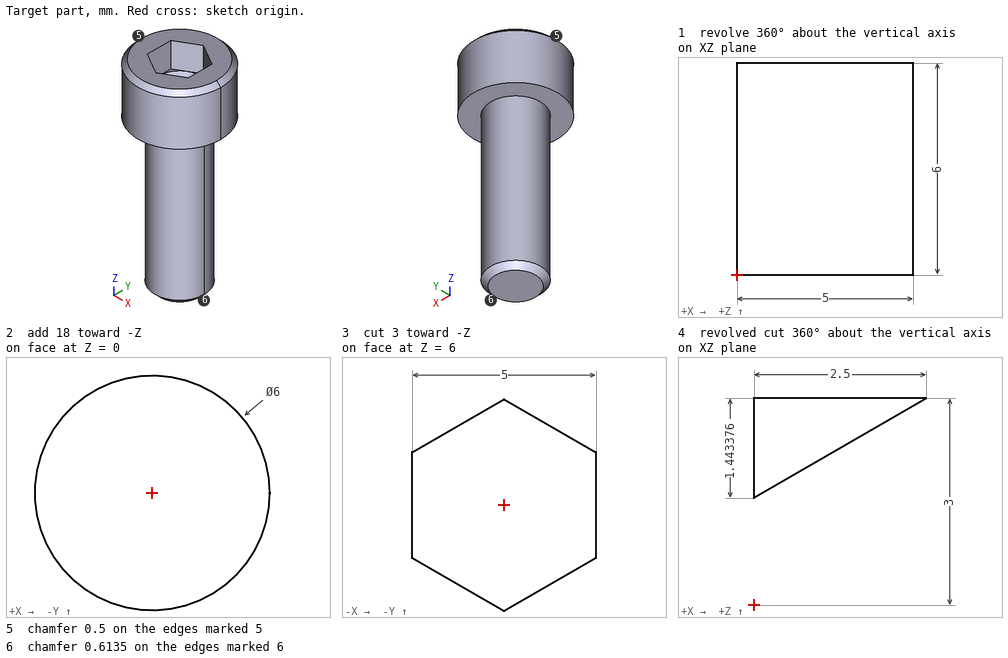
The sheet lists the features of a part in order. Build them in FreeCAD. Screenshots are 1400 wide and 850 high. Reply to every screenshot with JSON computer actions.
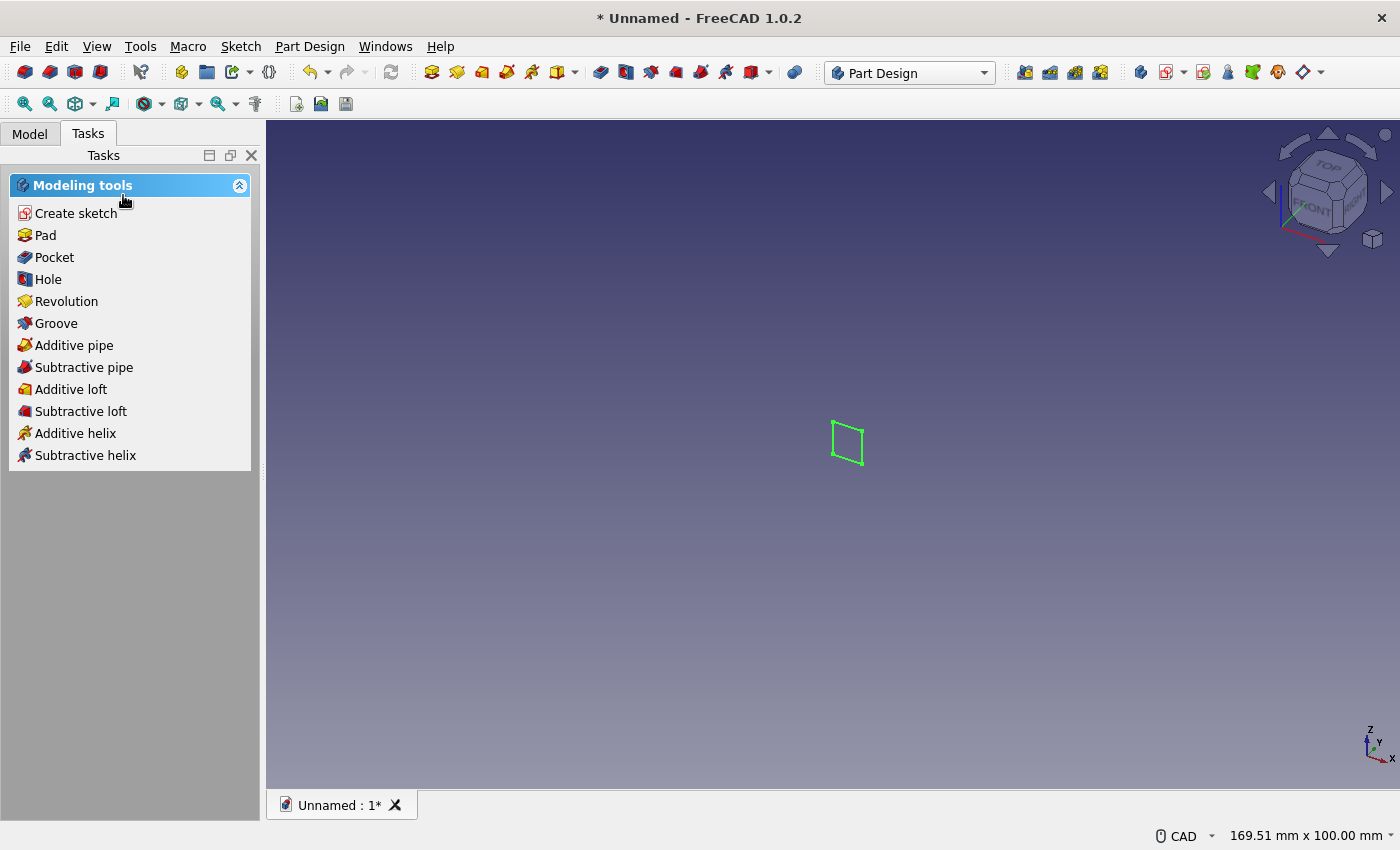
{"action": "left_click", "coordinate": [457, 72]}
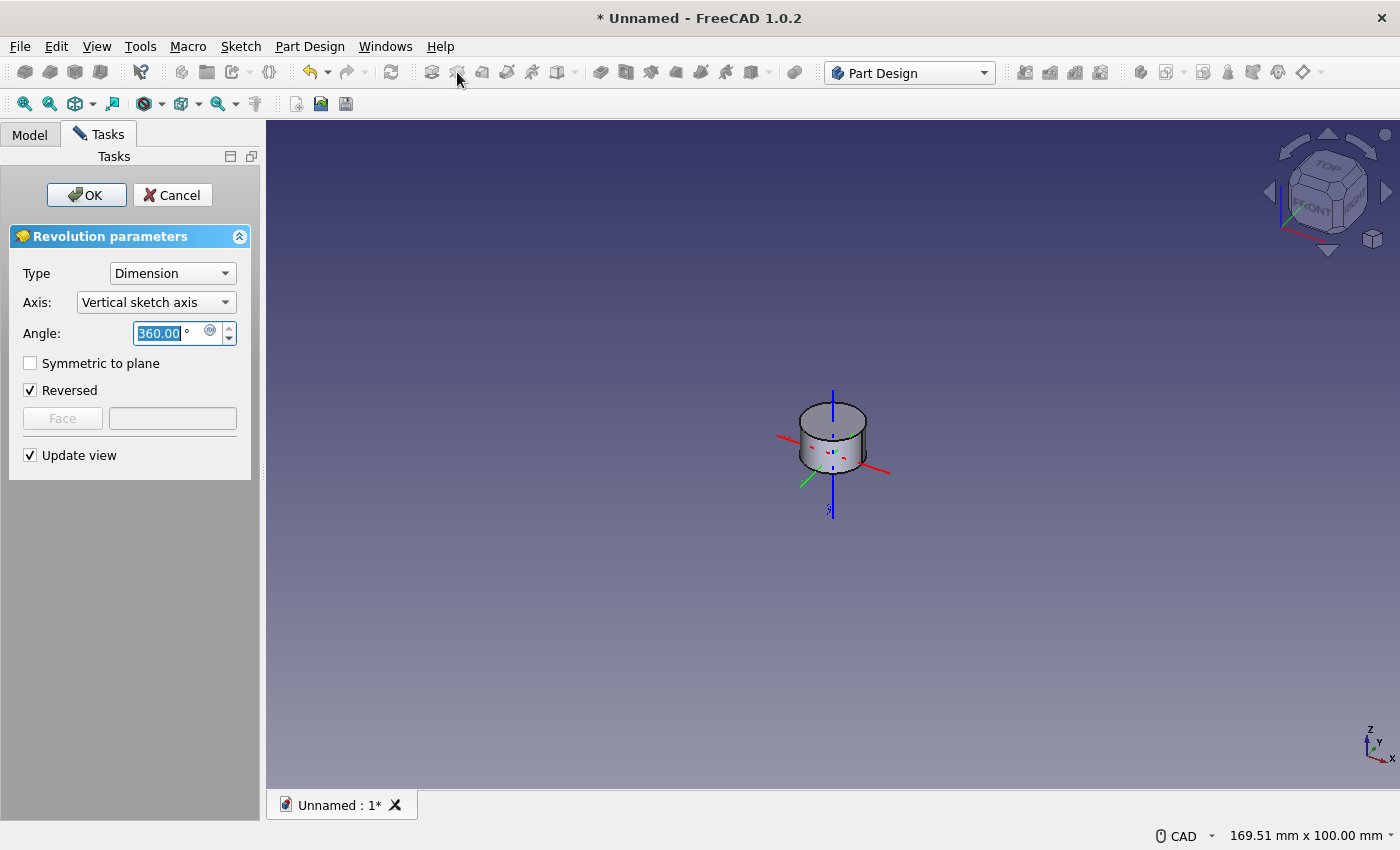
{"action": "left_click", "coordinate": [87, 195]}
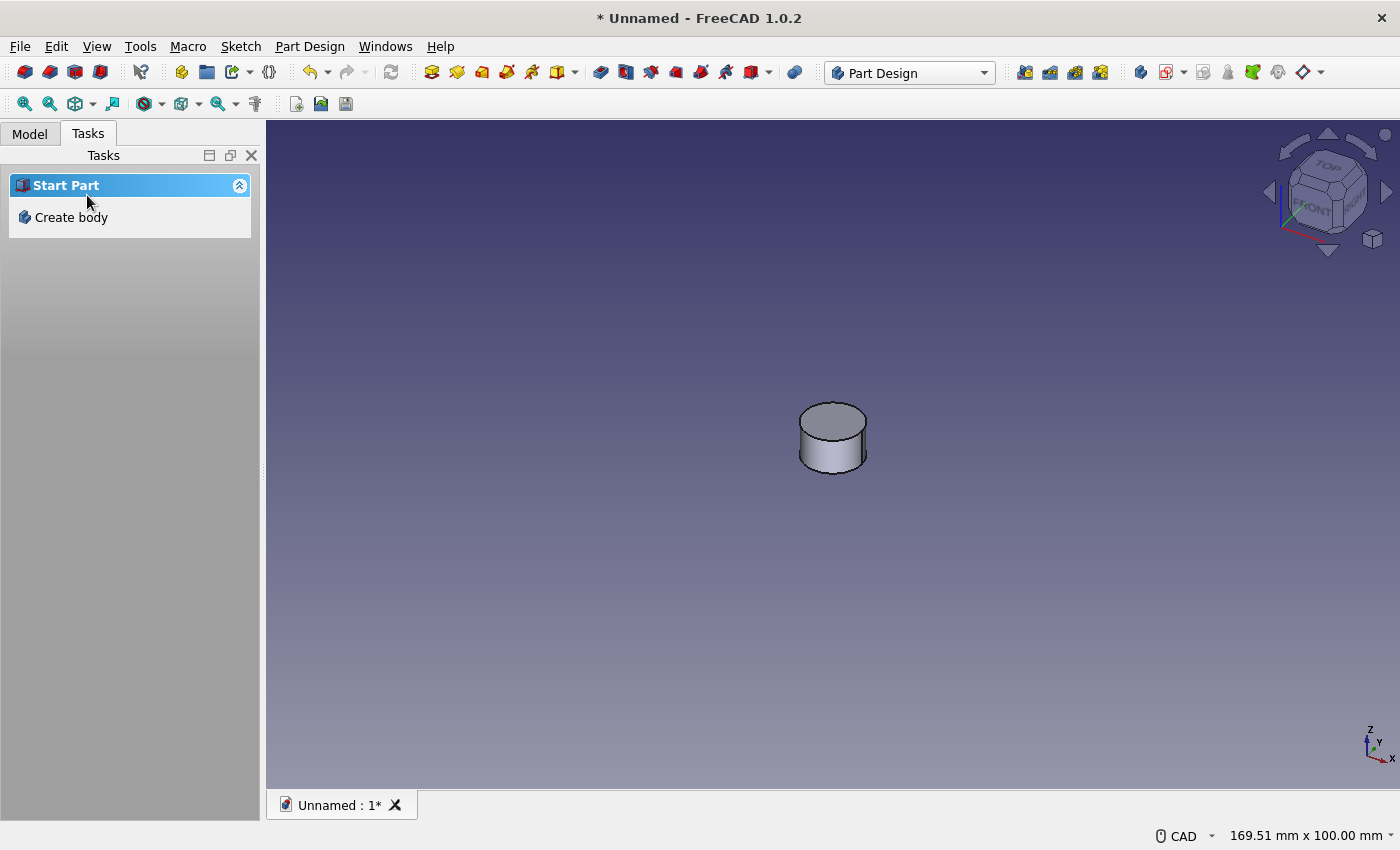
{"action": "left_click", "coordinate": [25, 104]}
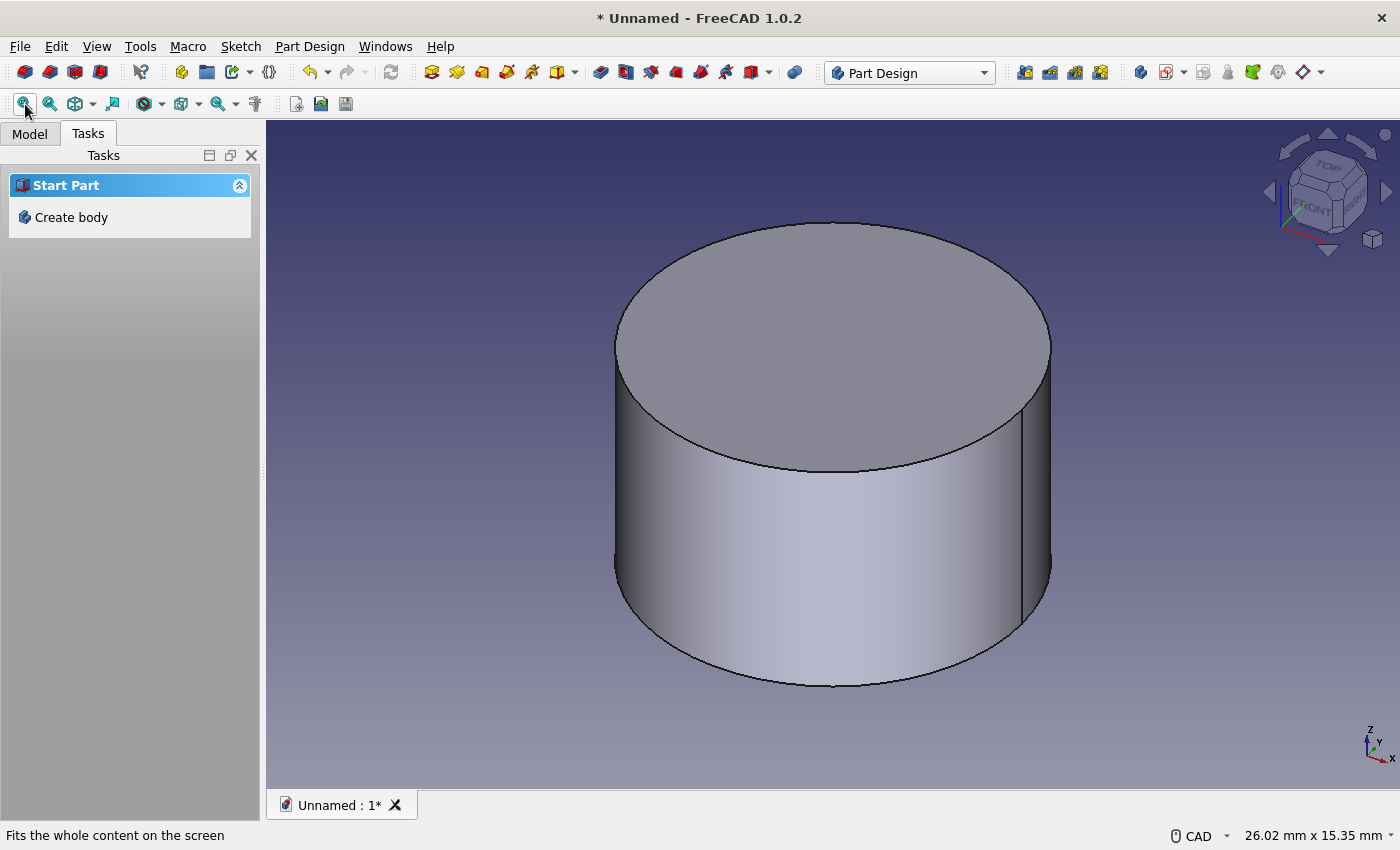
{"action": "key", "text": "5"}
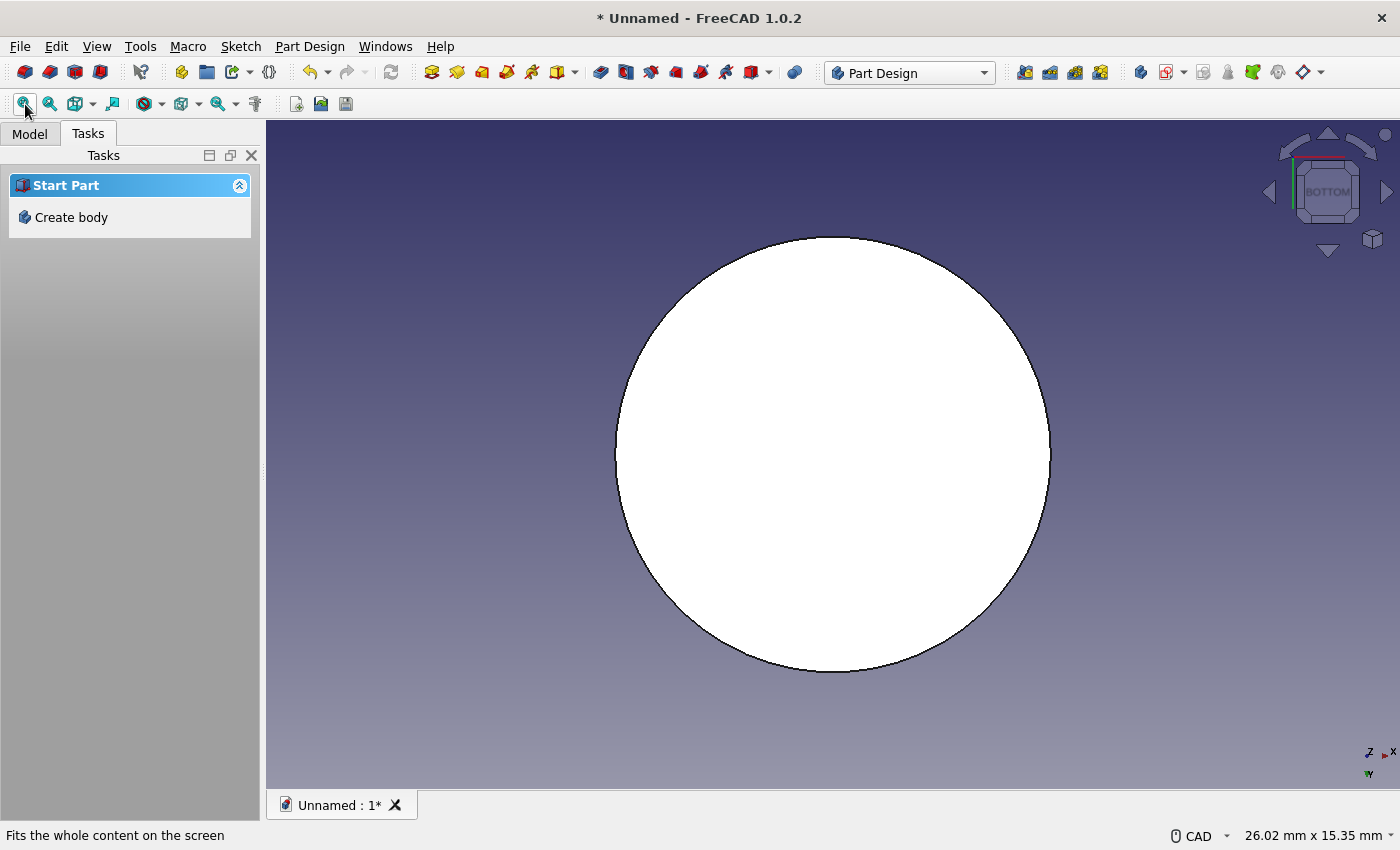
{"action": "left_click", "coordinate": [833, 454]}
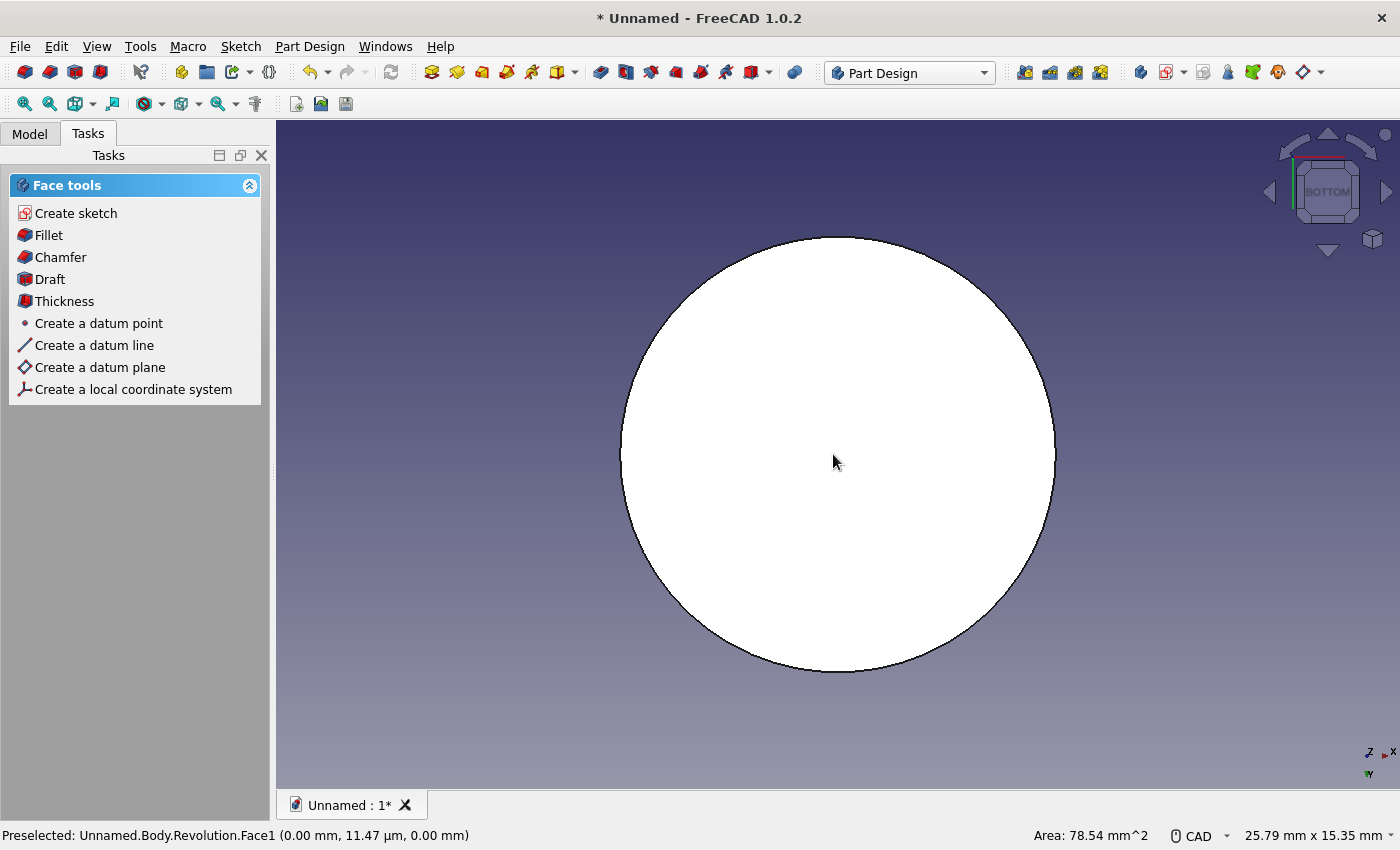
{"action": "left_click", "coordinate": [1166, 72]}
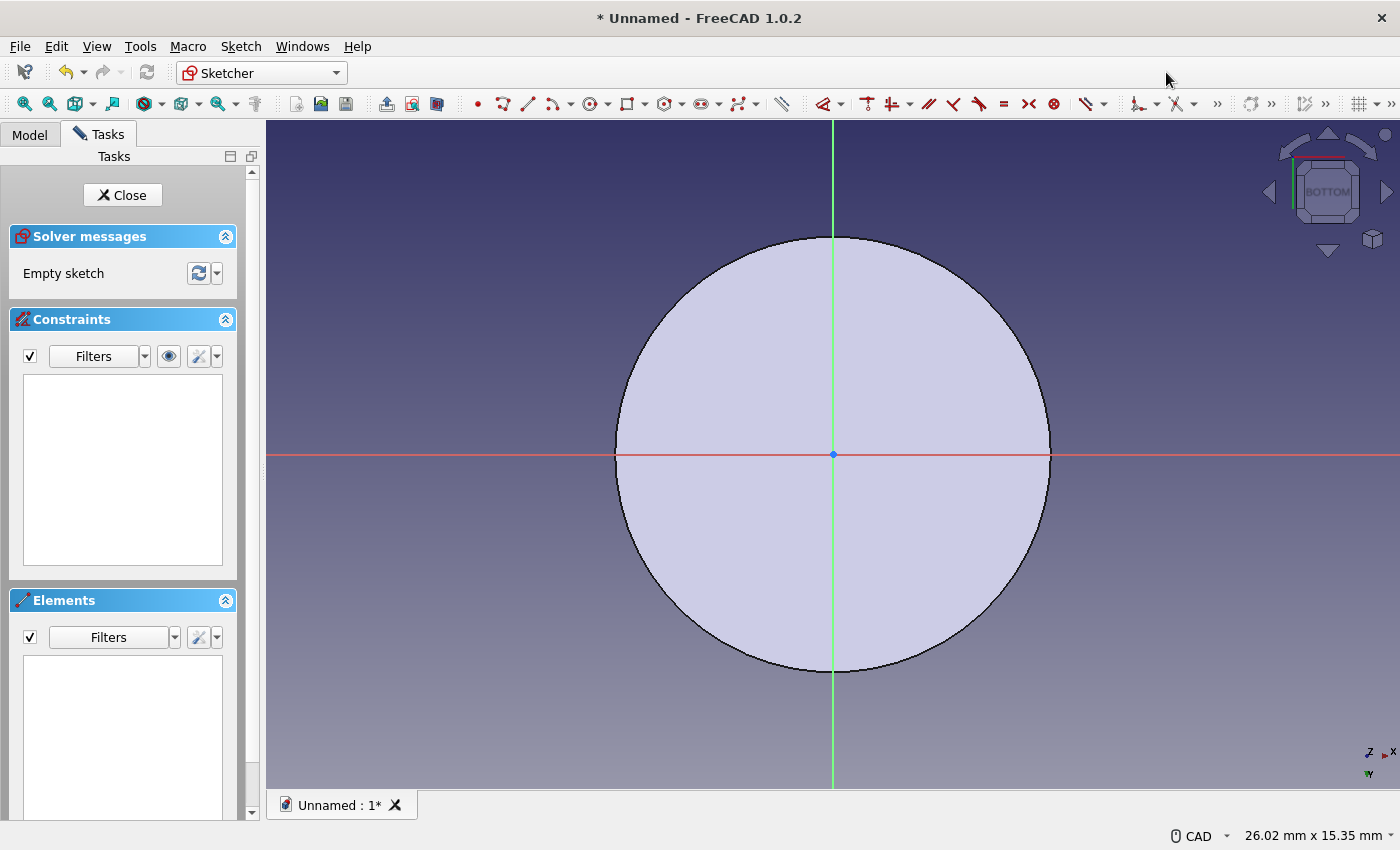
{"action": "scroll", "coordinate": [916, 455], "scroll_direction": "up", "scroll_amount": 3}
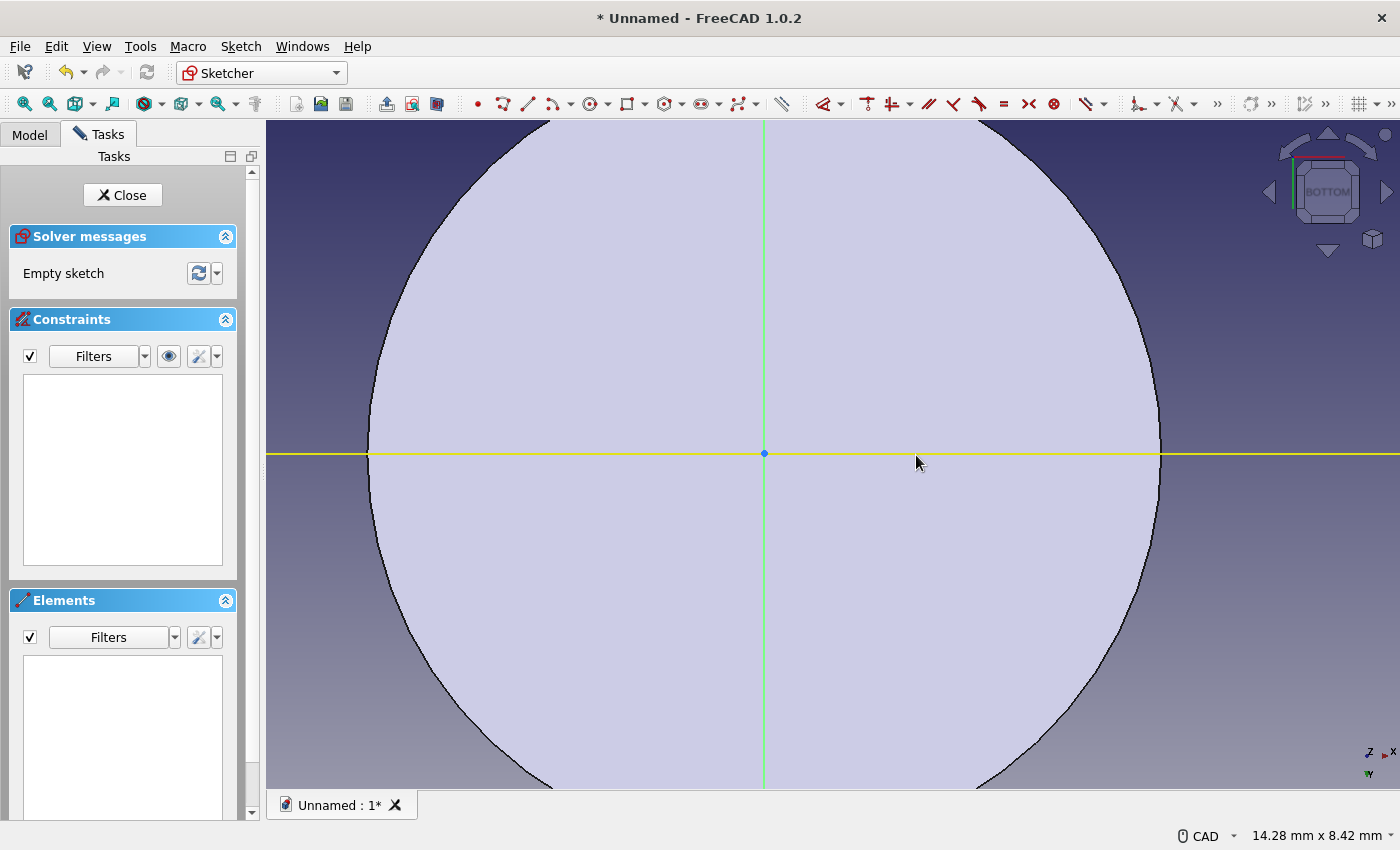
{"action": "left_click", "coordinate": [590, 104]}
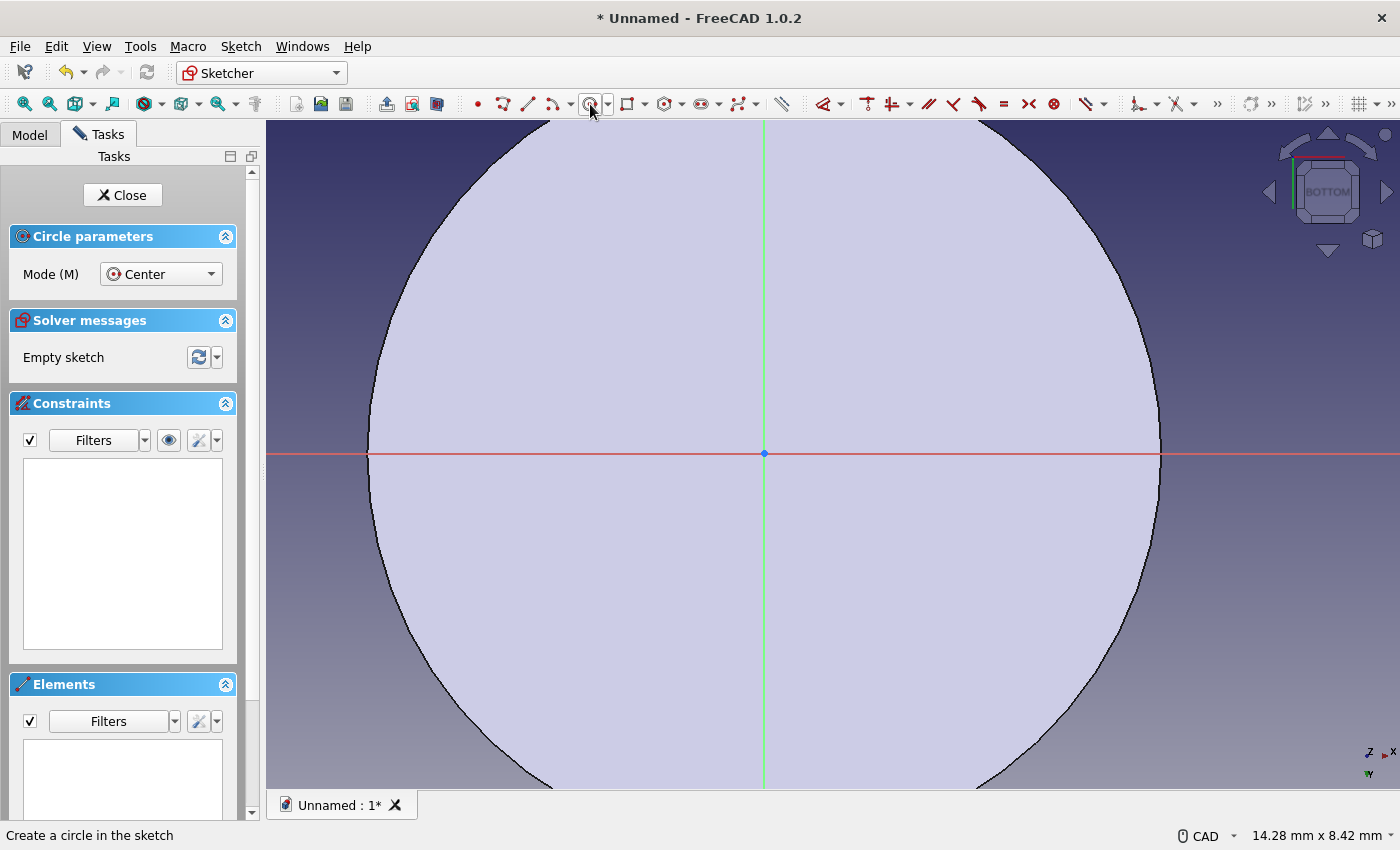
{"action": "left_click", "coordinate": [764, 454]}
{"action": "mouse_move", "coordinate": [933, 285]}